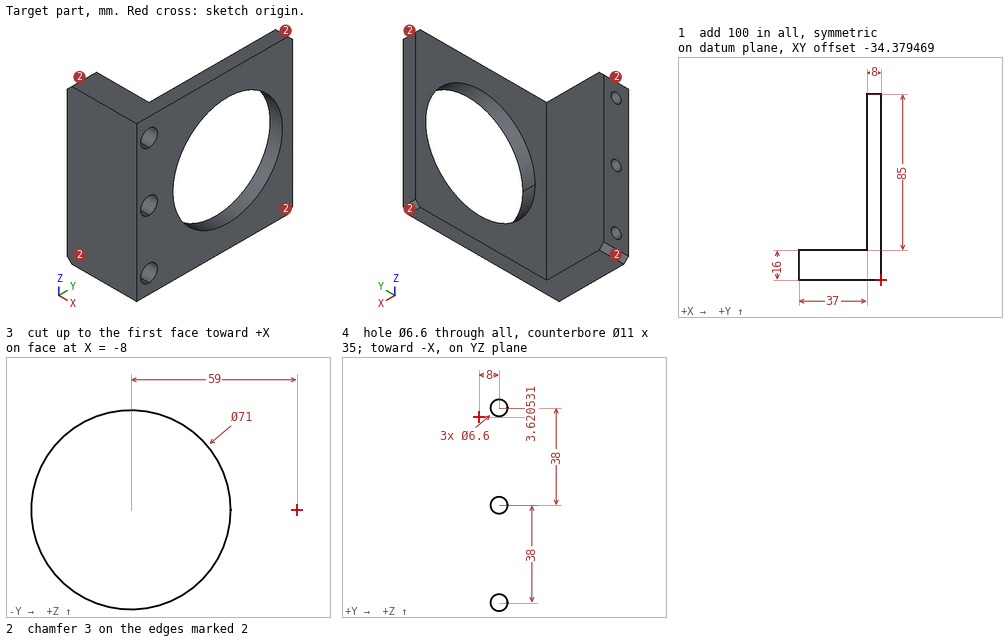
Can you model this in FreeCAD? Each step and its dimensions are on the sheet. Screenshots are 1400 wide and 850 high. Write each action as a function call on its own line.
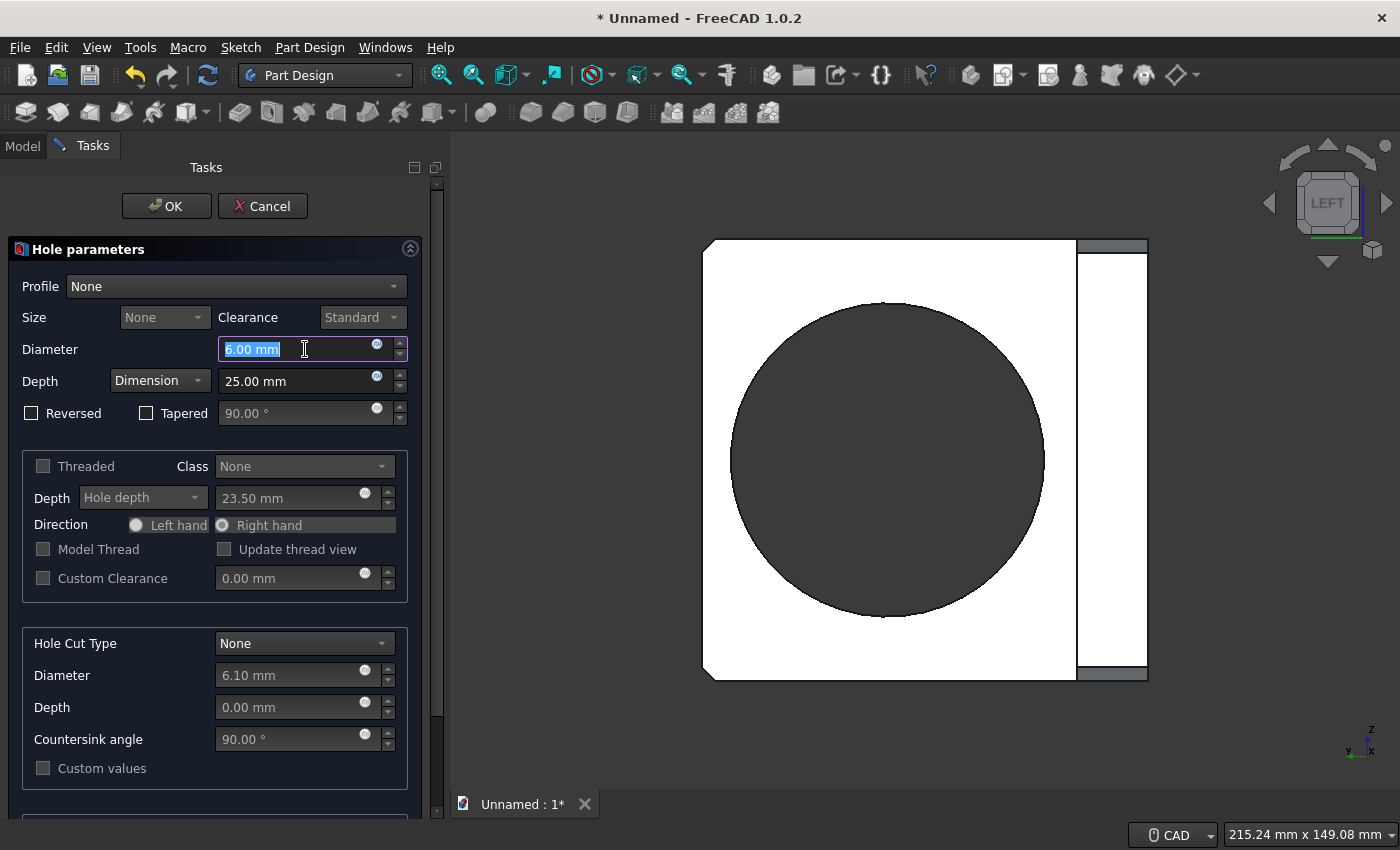
text(6.6)
key(Tab)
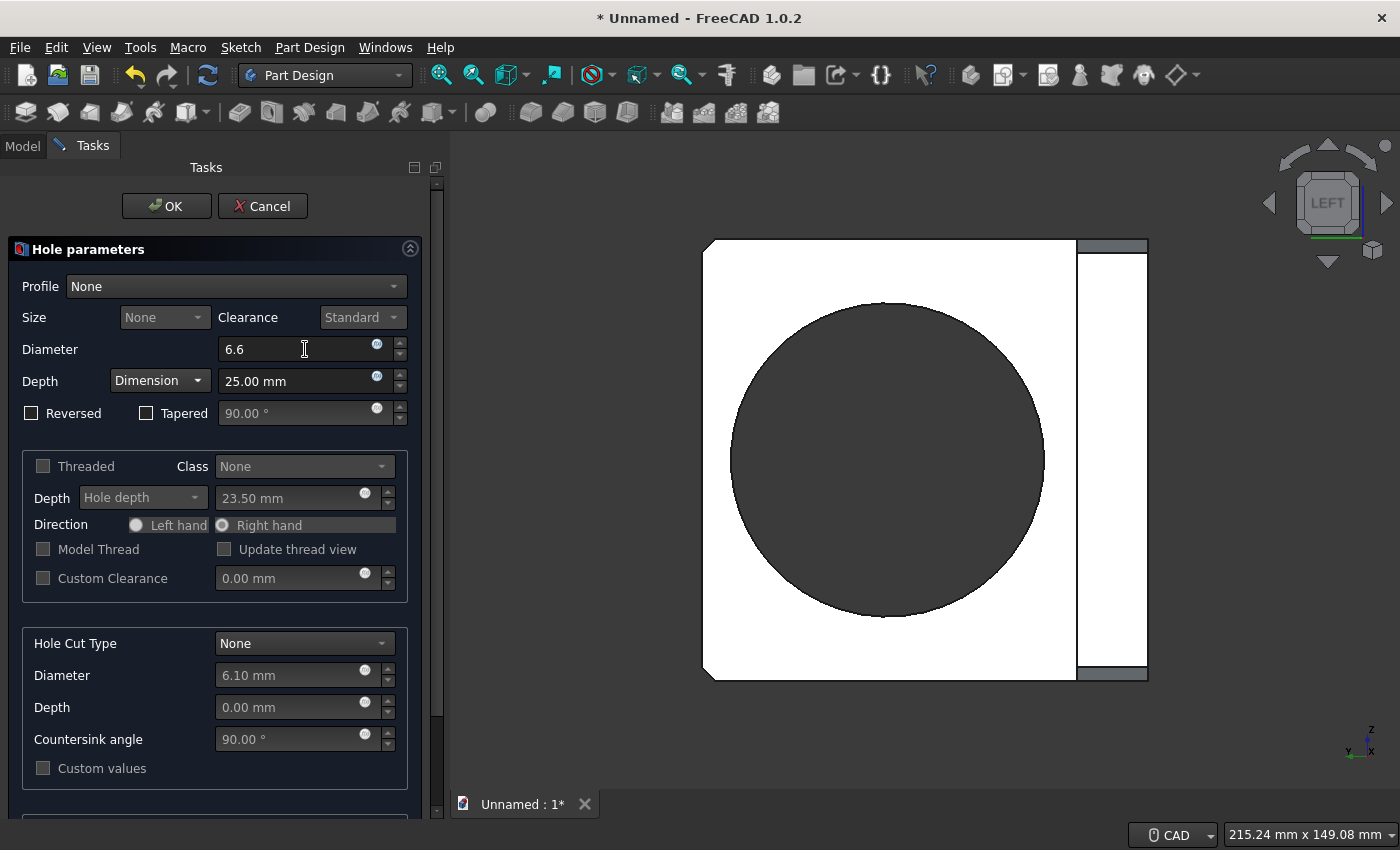
click(161, 380)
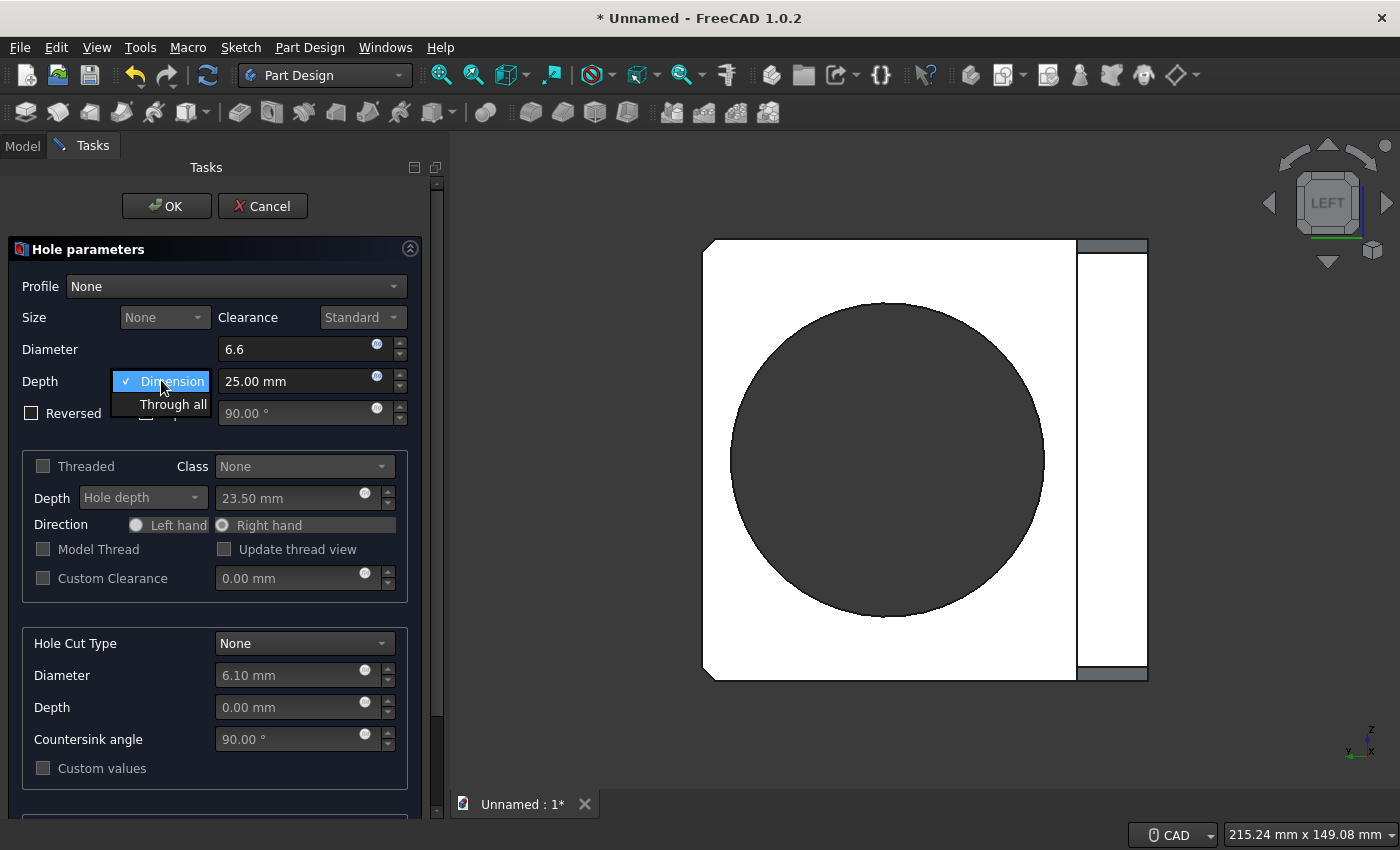
click(160, 404)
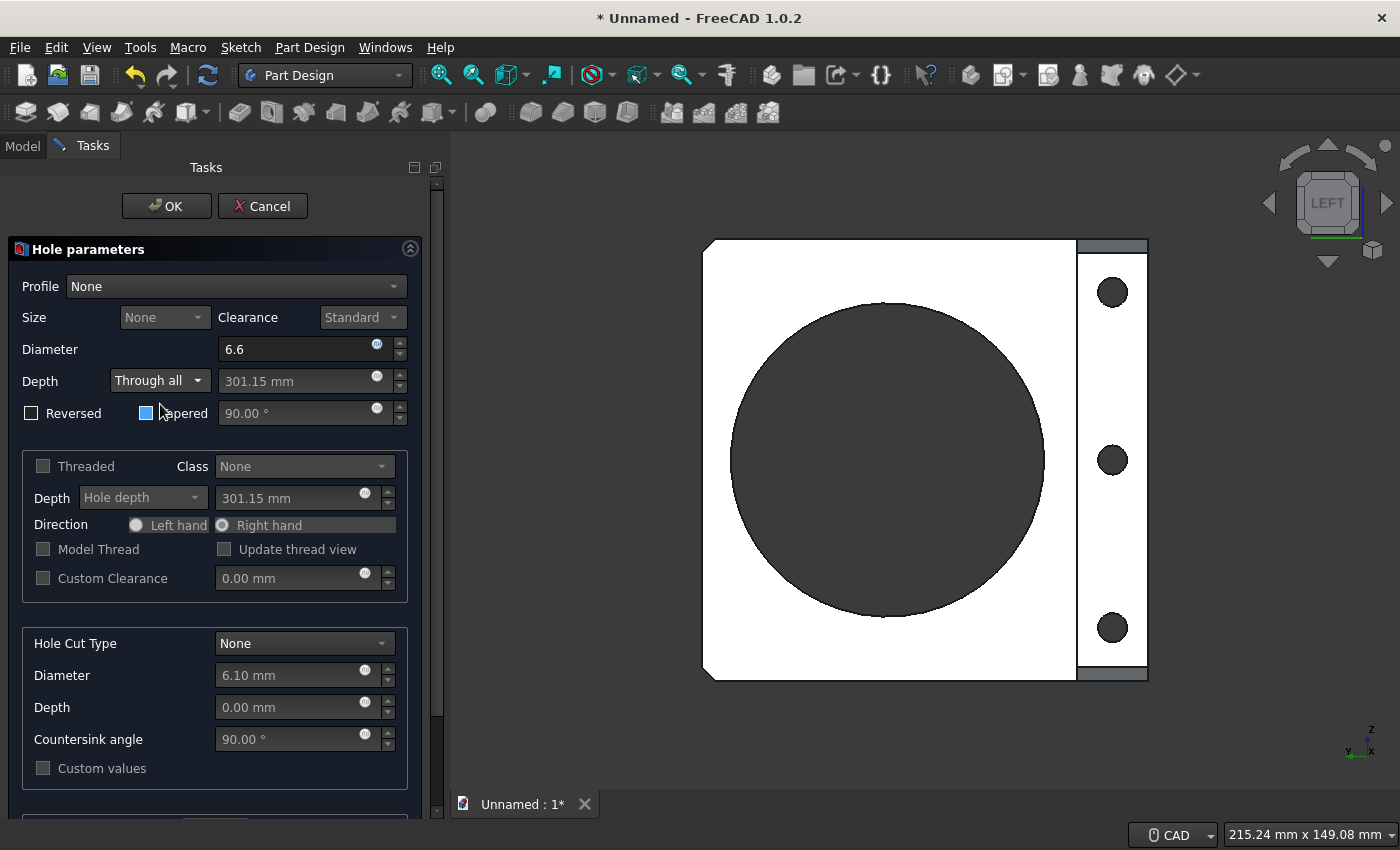
click(306, 644)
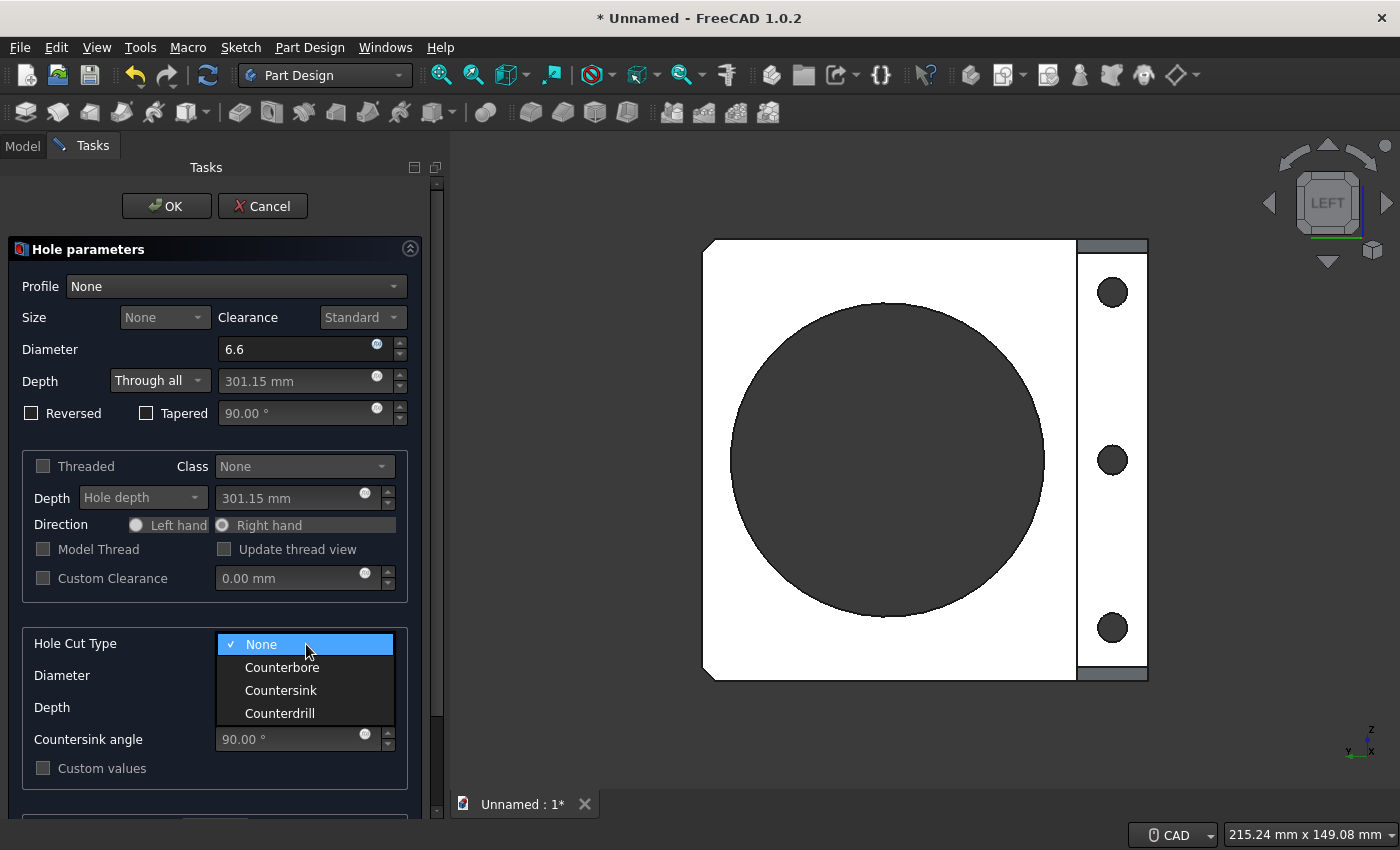
click(304, 668)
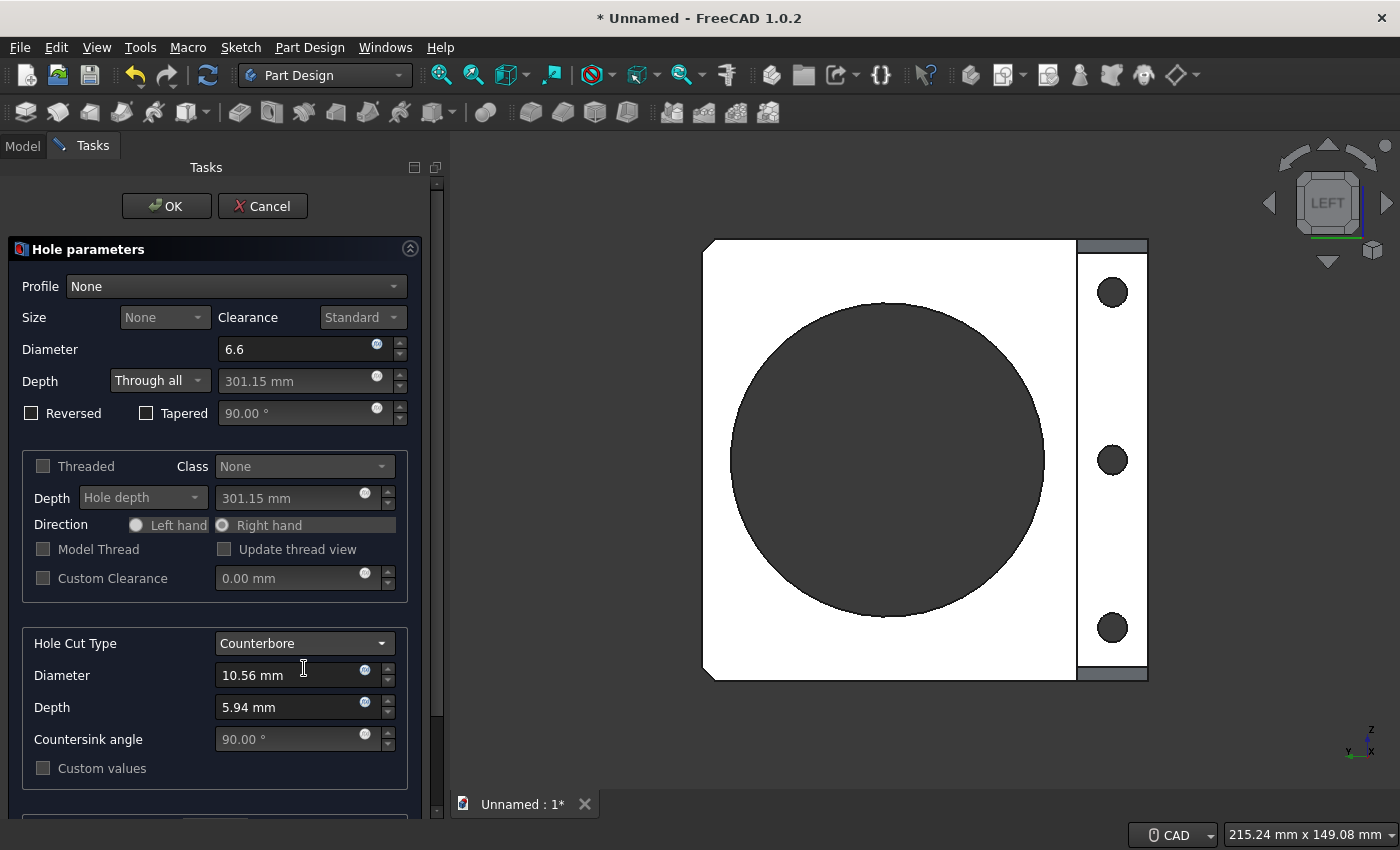
triple_click(298, 675)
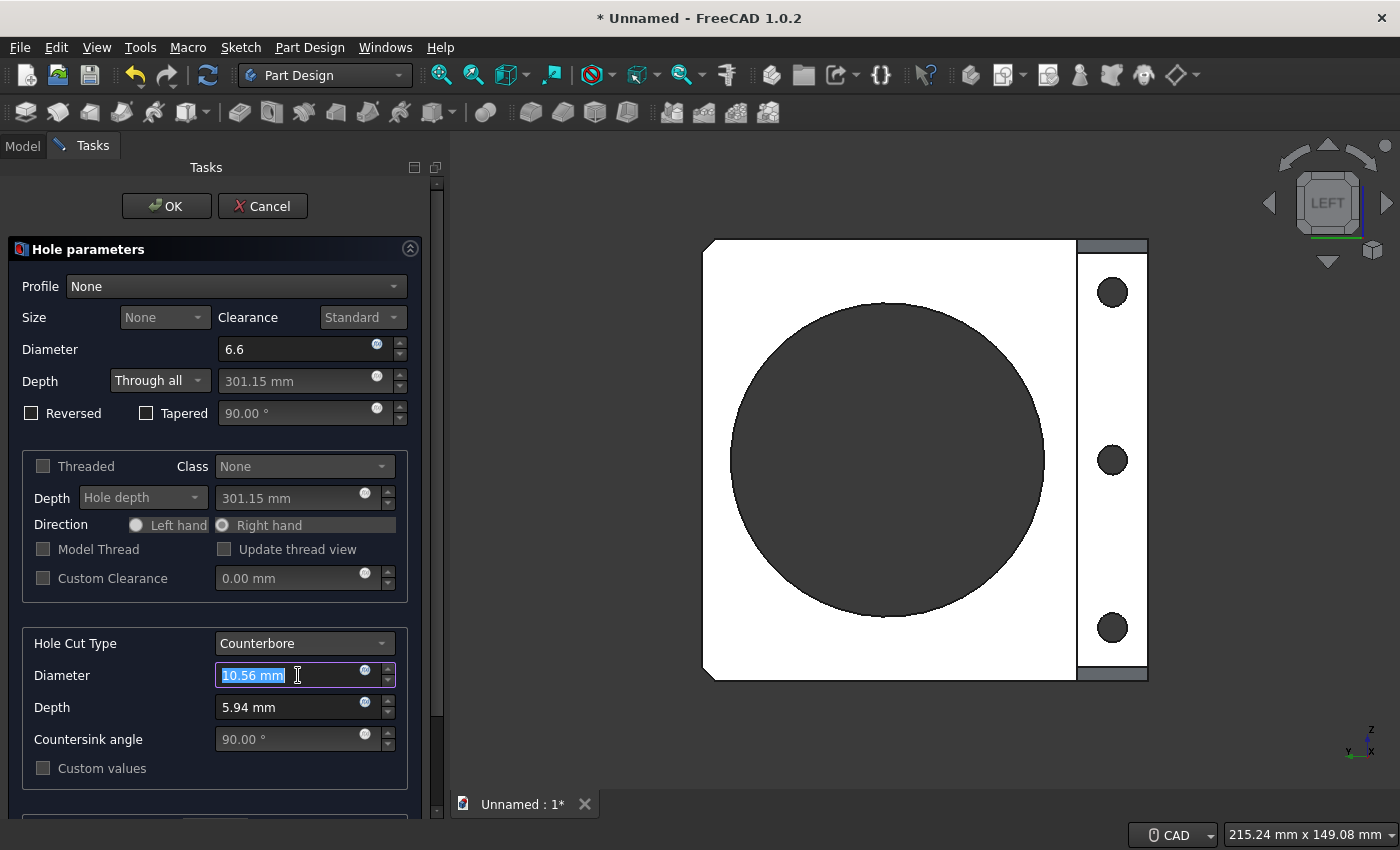
text(11)
key(Tab)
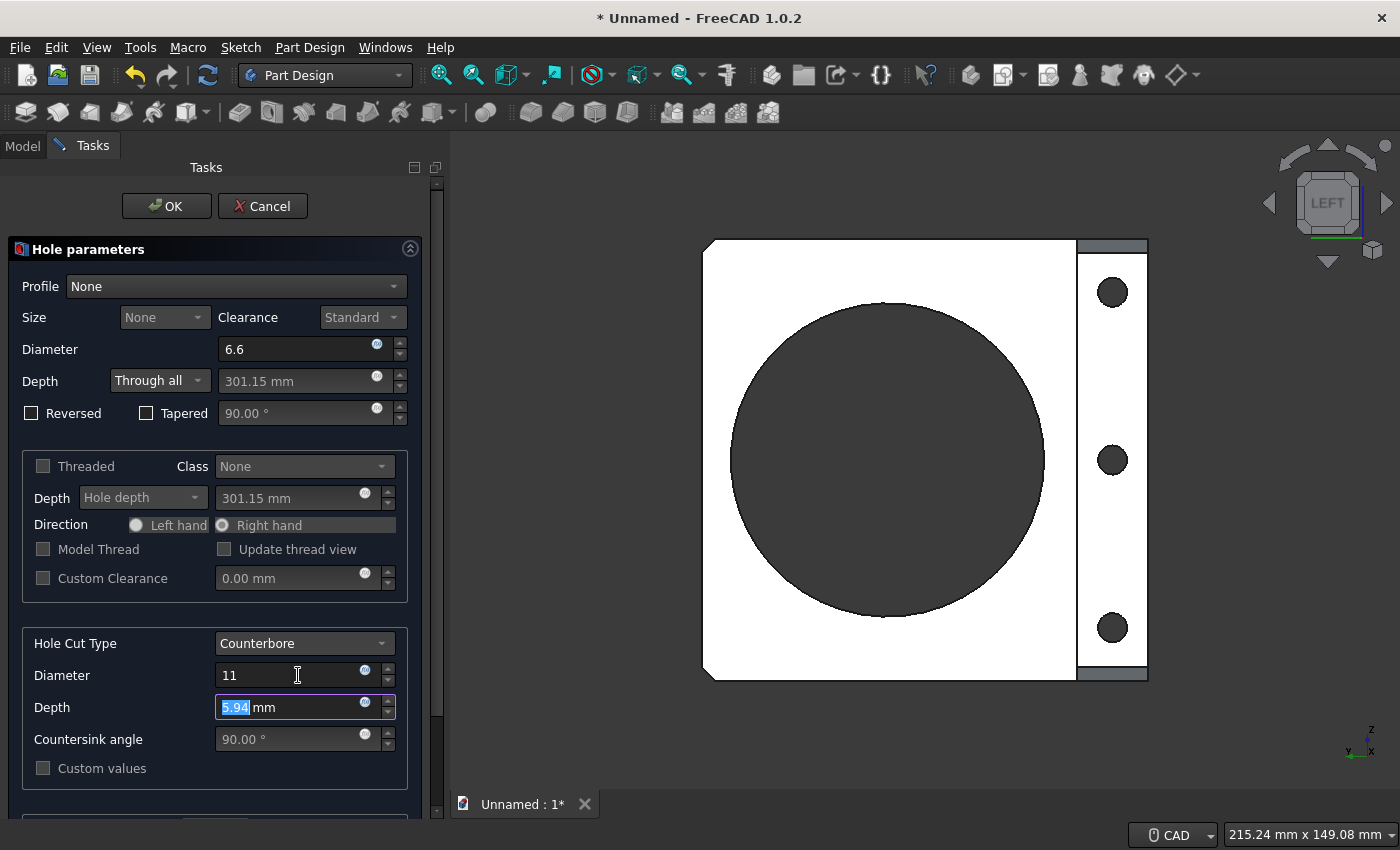
text(35)
key(Tab)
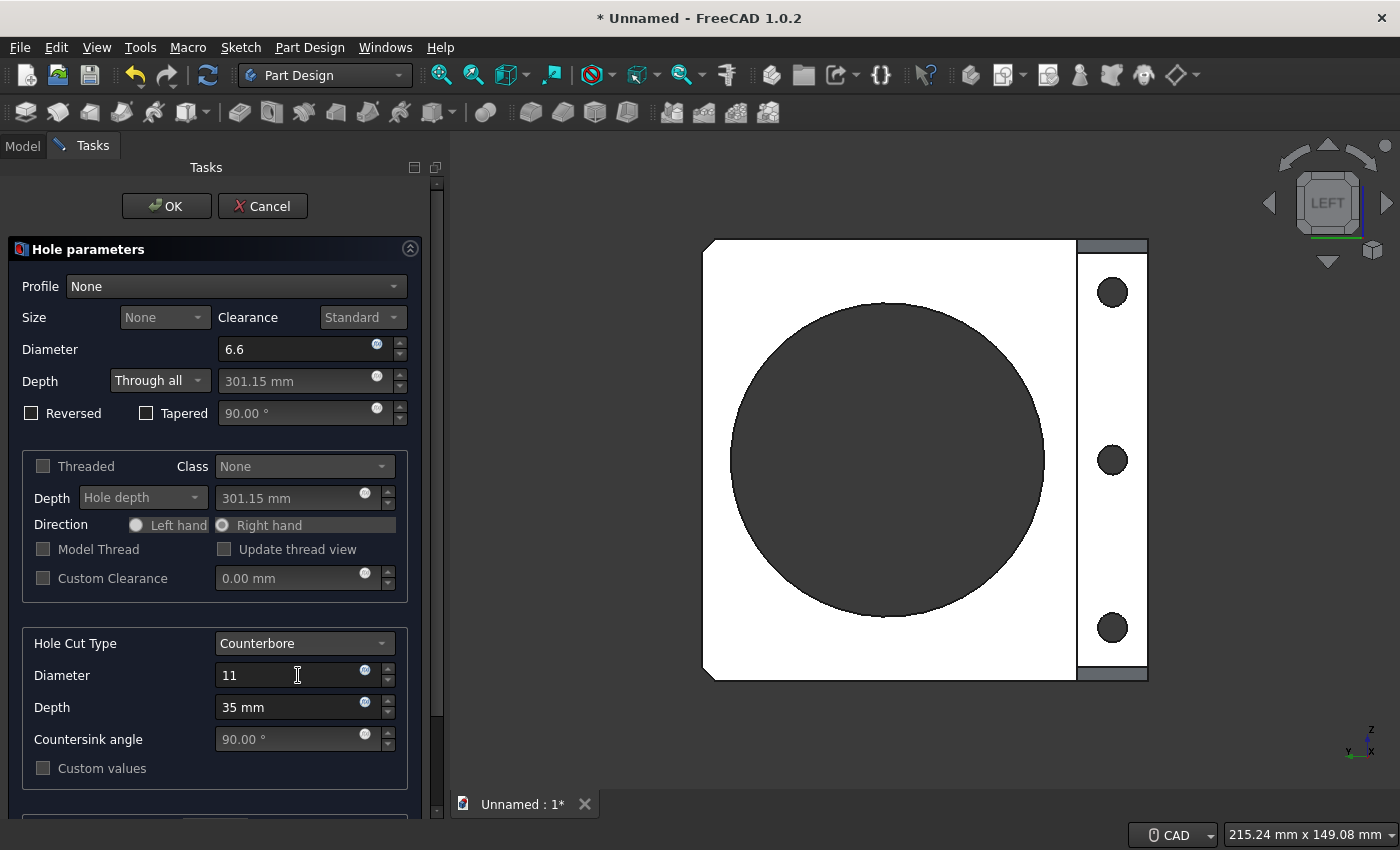
click(167, 206)